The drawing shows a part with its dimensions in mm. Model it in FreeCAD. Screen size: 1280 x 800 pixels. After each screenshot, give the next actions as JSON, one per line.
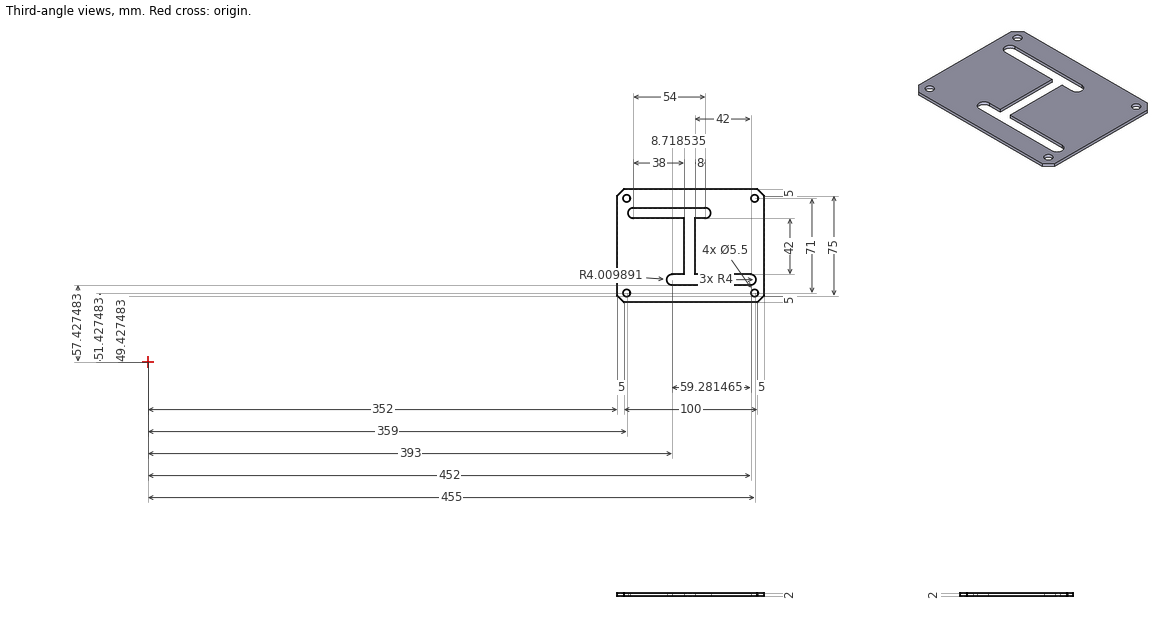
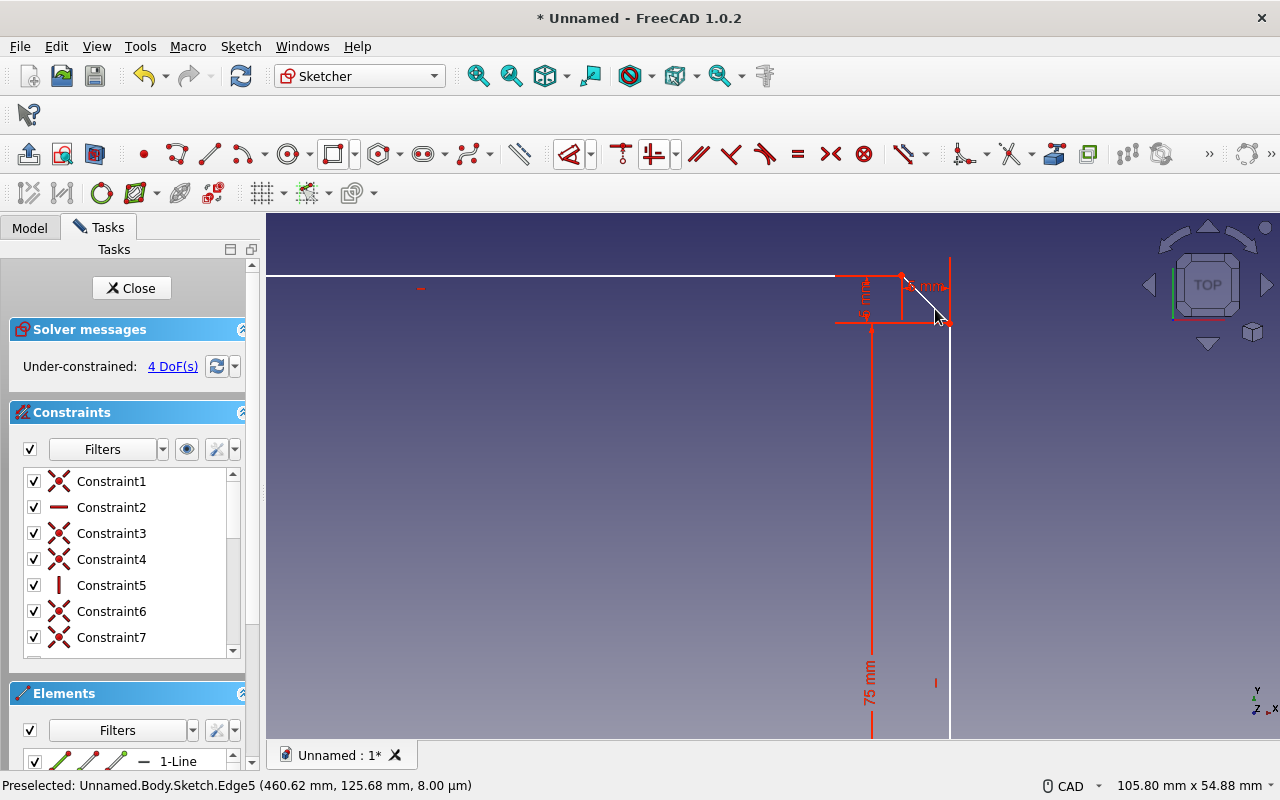
{"action": "scroll", "coordinate": [935, 309], "scroll_direction": "down", "scroll_amount": 4}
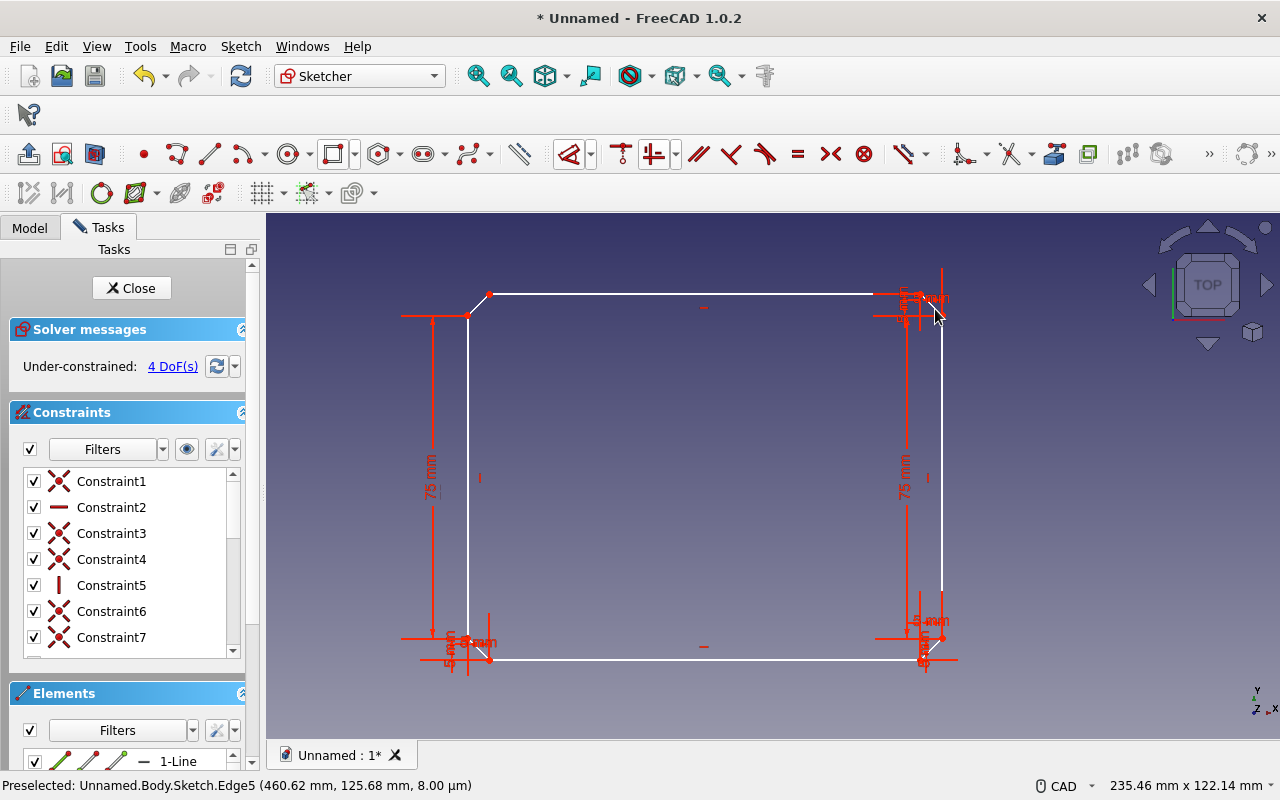
{"action": "scroll", "coordinate": [483, 301], "scroll_direction": "up", "scroll_amount": 4}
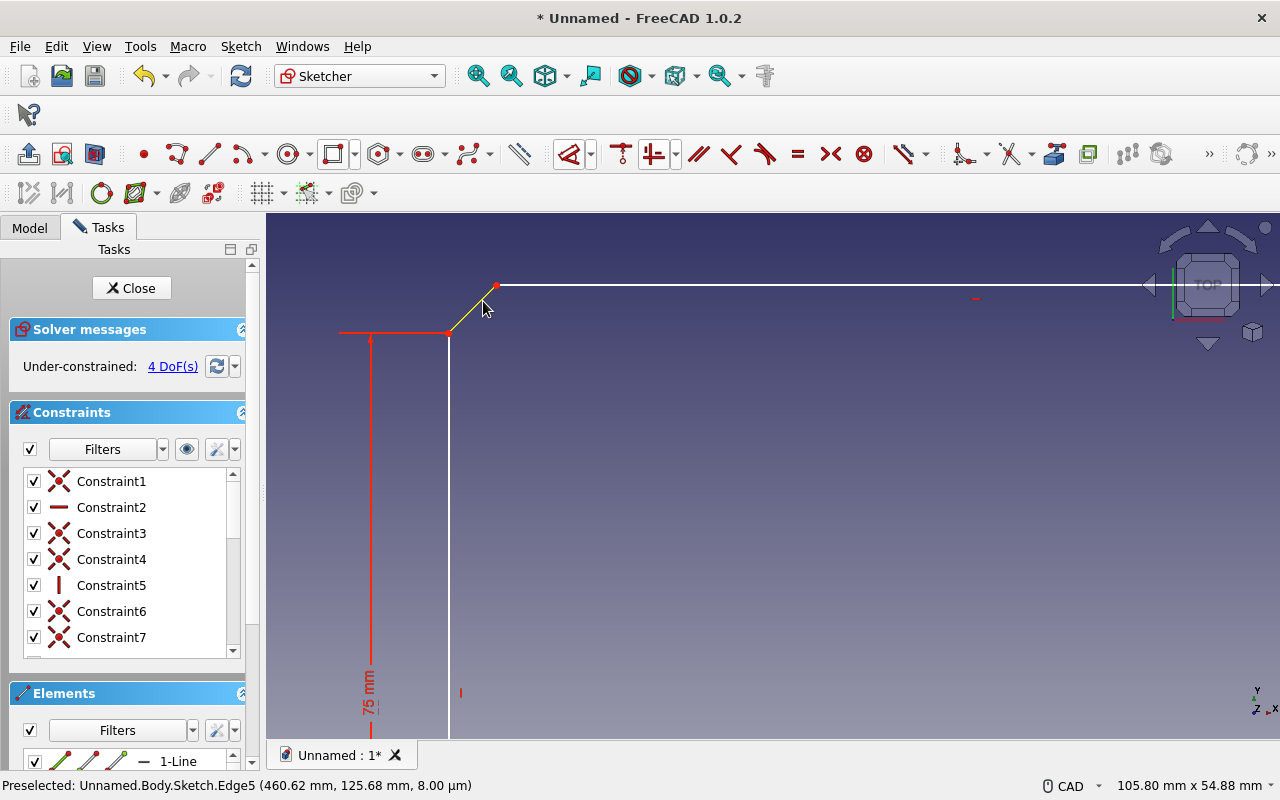
{"action": "left_click", "coordinate": [482, 300]}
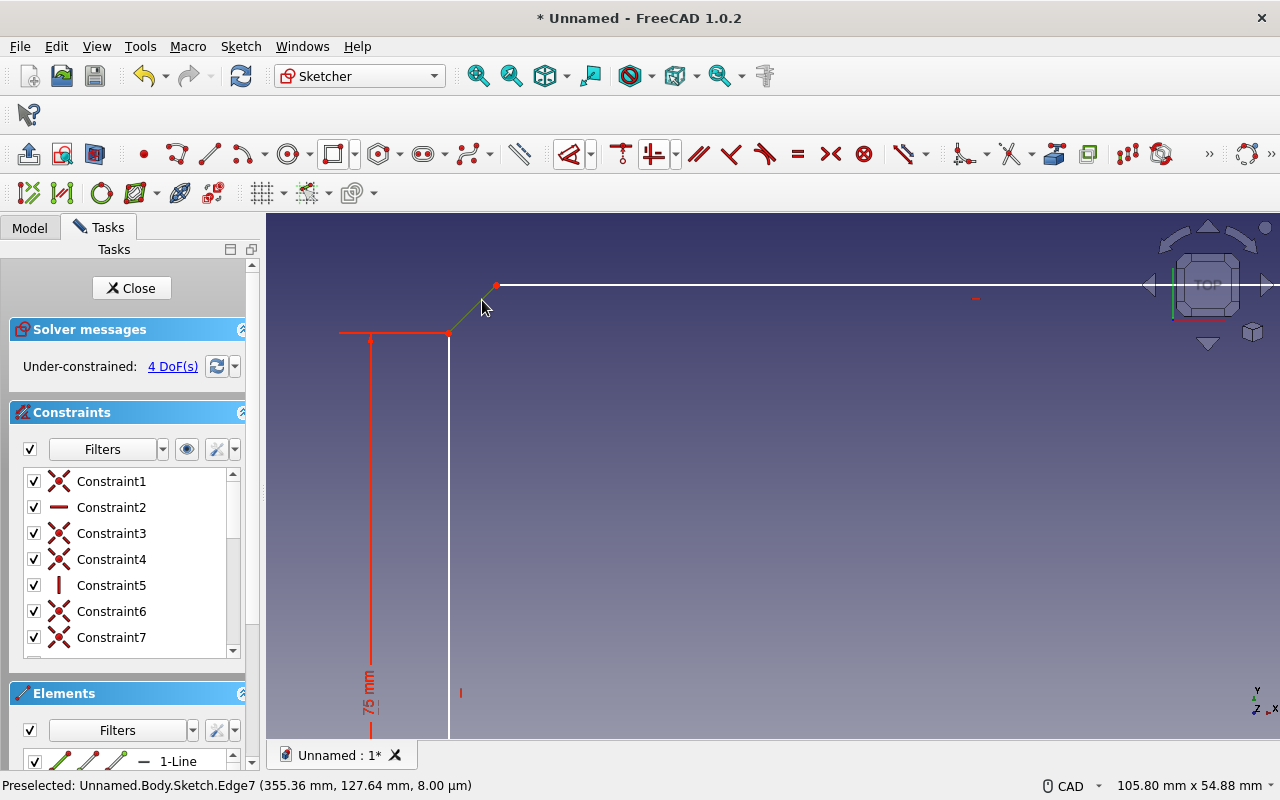
{"action": "left_click", "coordinate": [590, 154]}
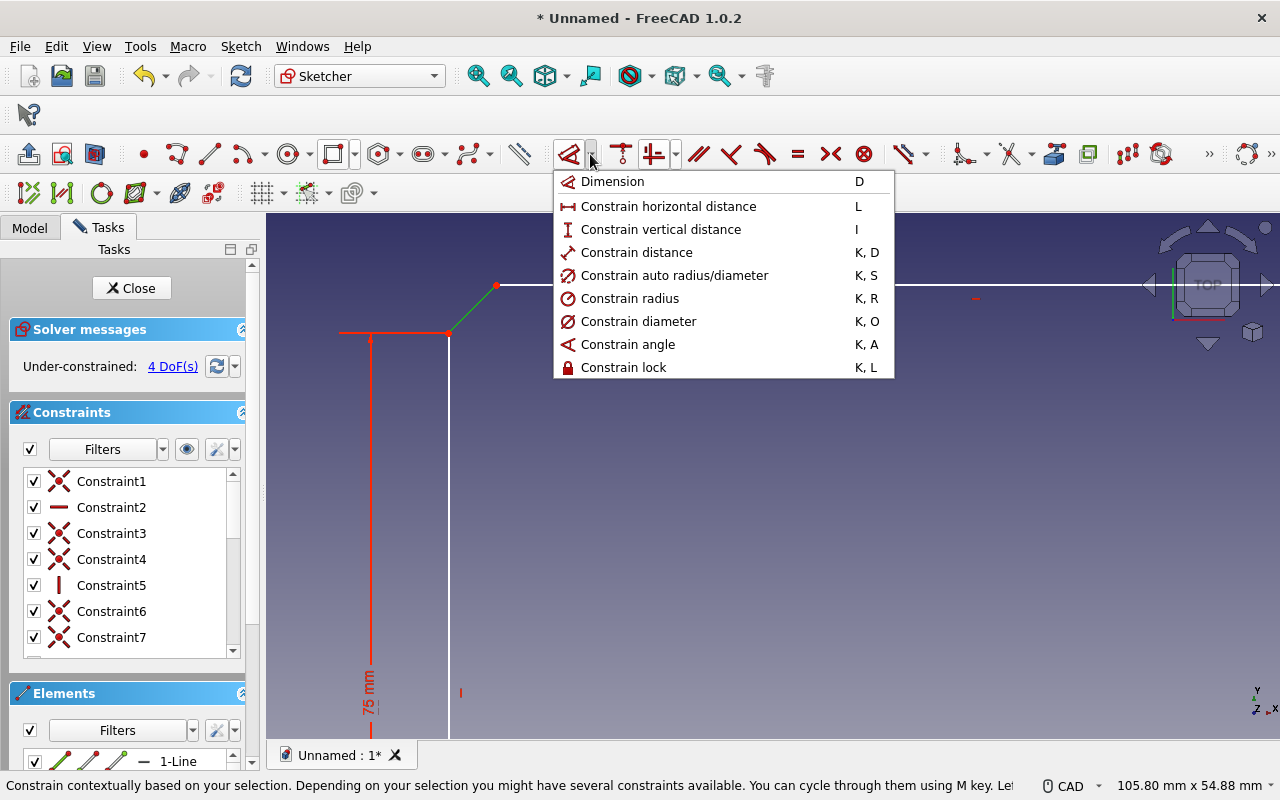
{"action": "left_click", "coordinate": [724, 206]}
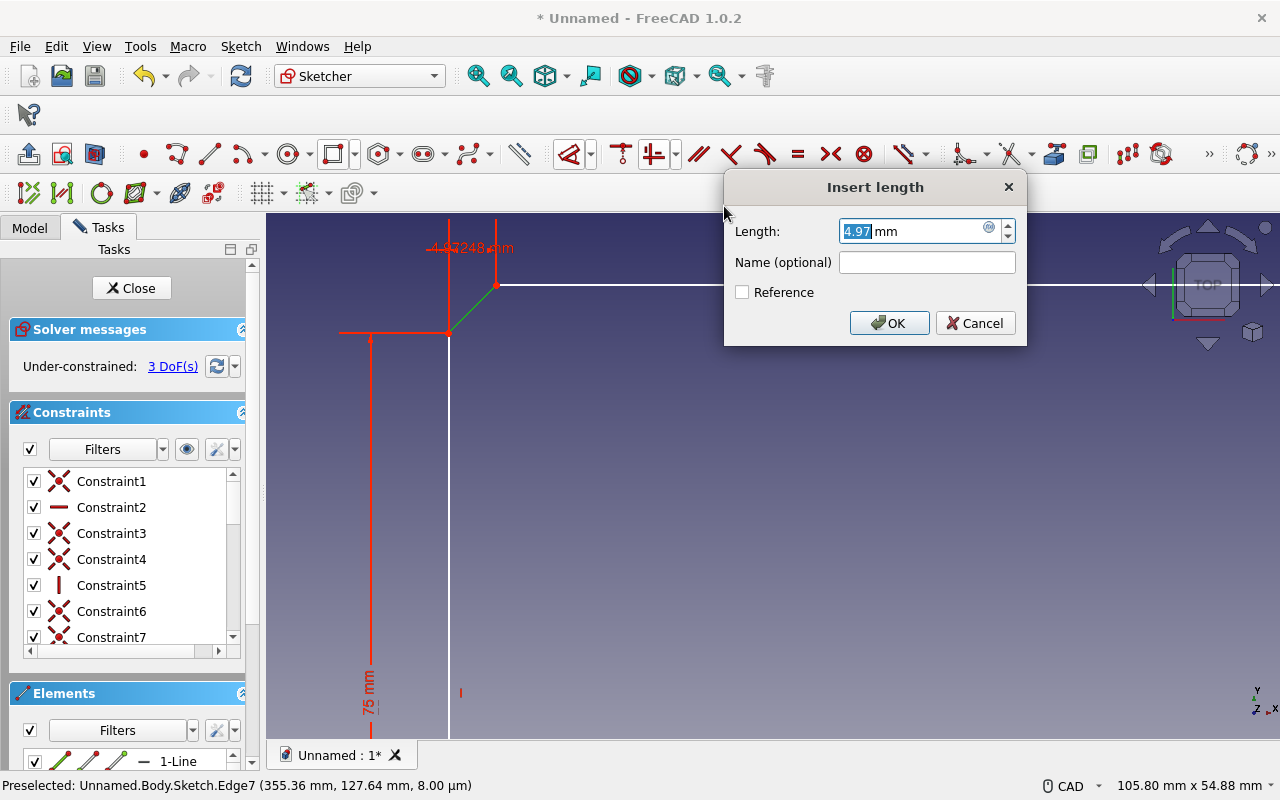
{"action": "type", "text": "5"}
{"action": "key", "text": "Return"}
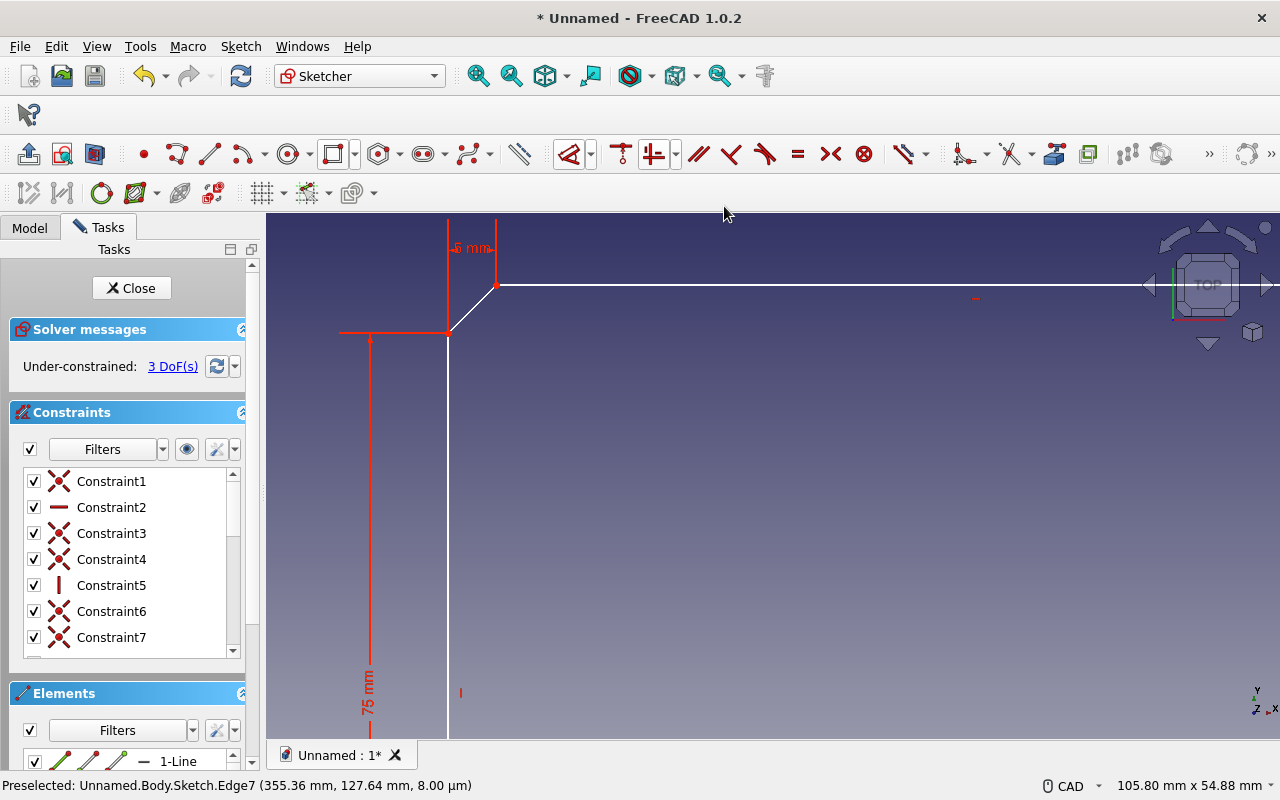
{"action": "scroll", "coordinate": [483, 301], "scroll_direction": "down", "scroll_amount": 4}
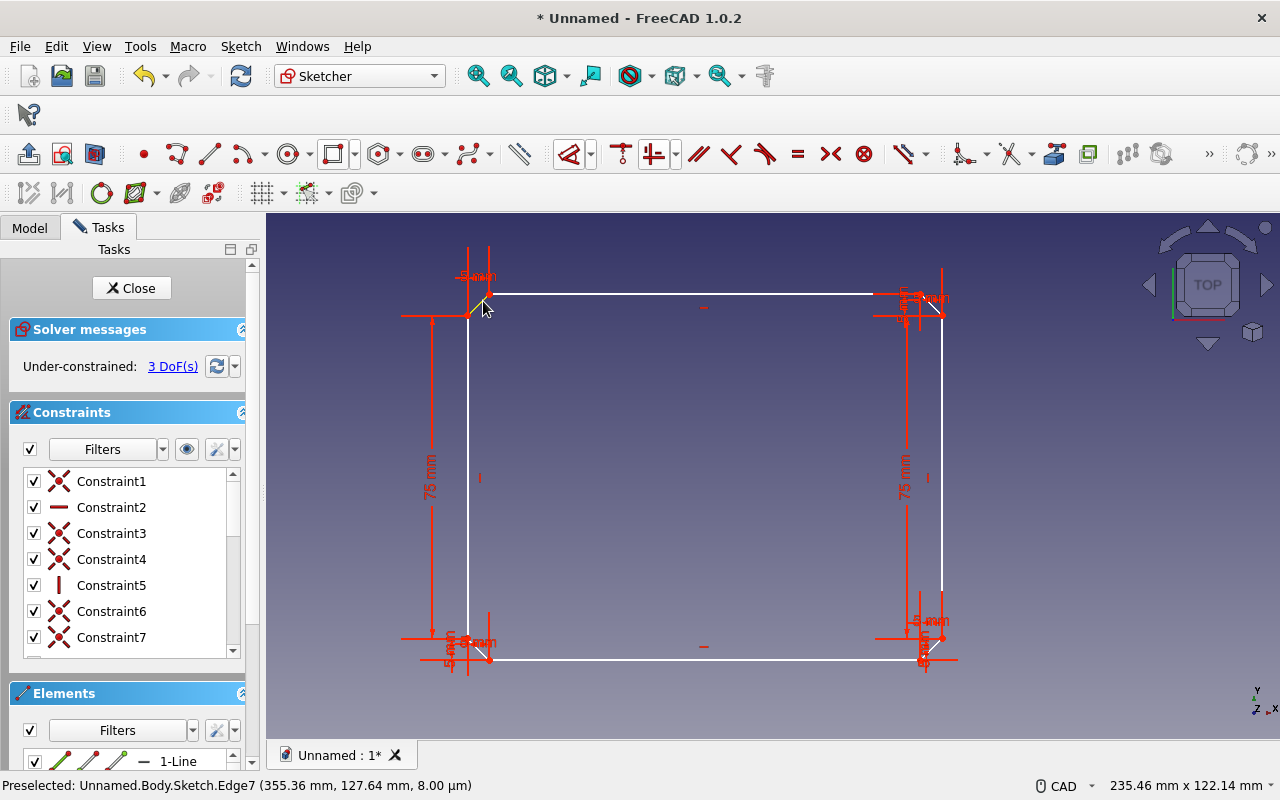
{"action": "left_click", "coordinate": [618, 660]}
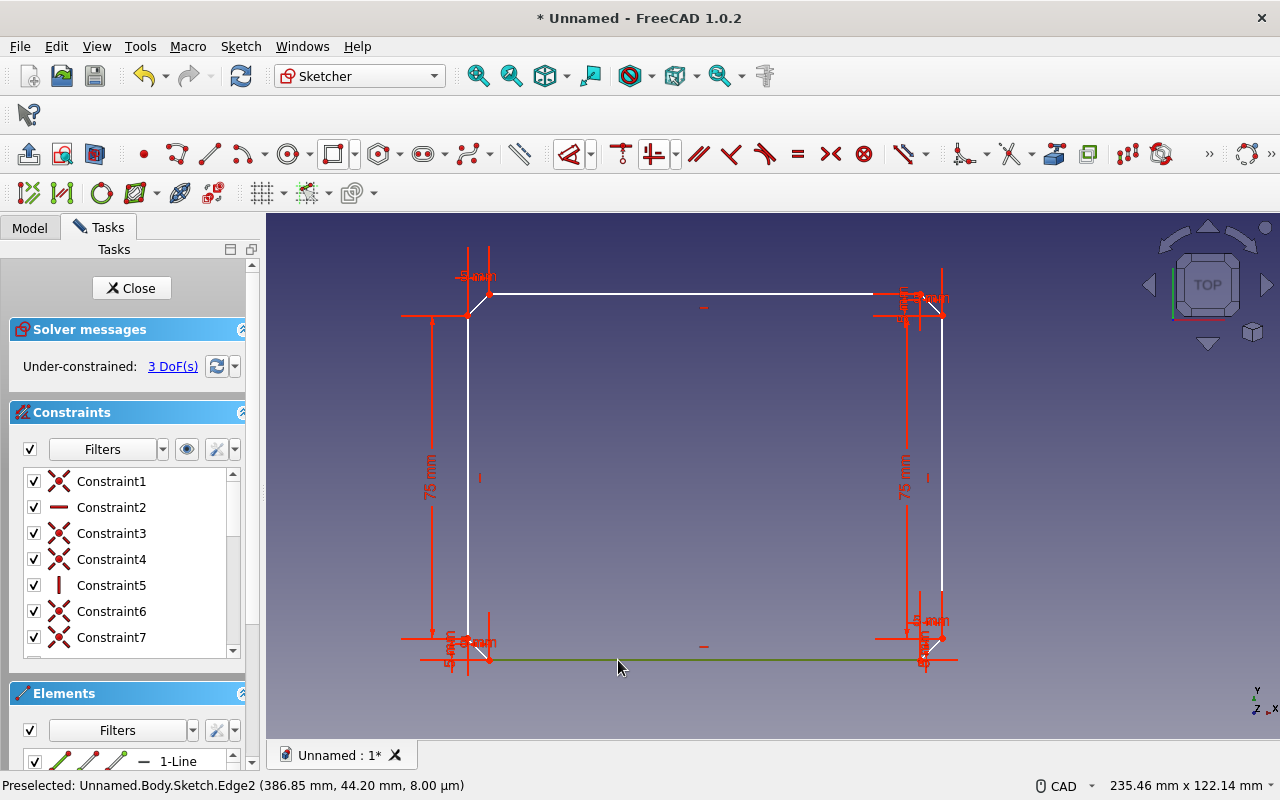
{"action": "key", "text": "l"}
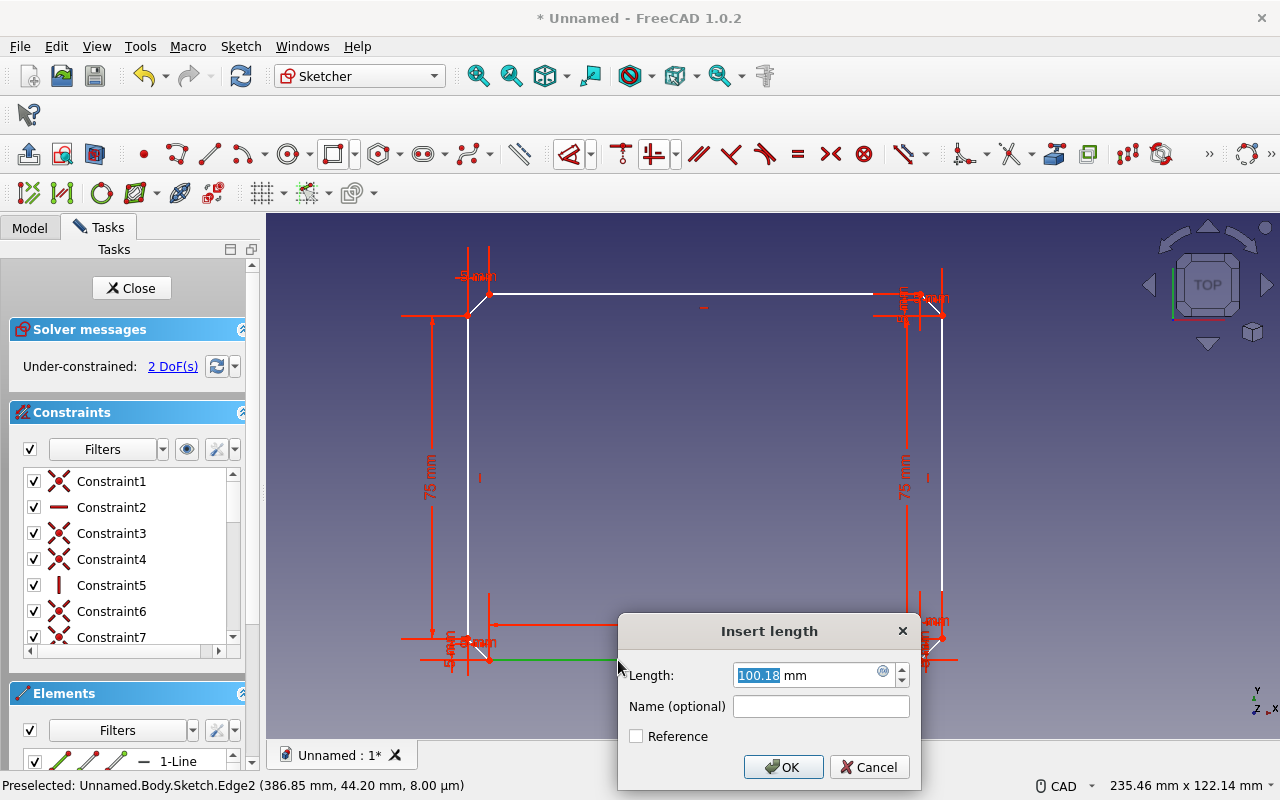
{"action": "type", "text": "100"}
{"action": "key", "text": "Return"}